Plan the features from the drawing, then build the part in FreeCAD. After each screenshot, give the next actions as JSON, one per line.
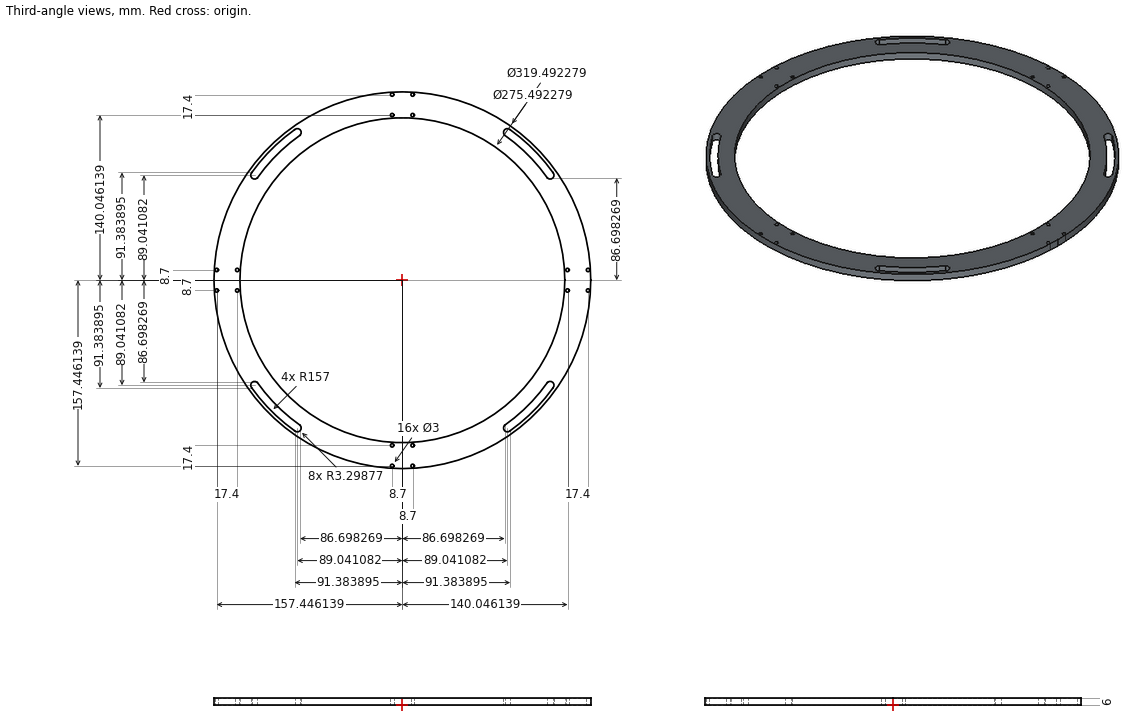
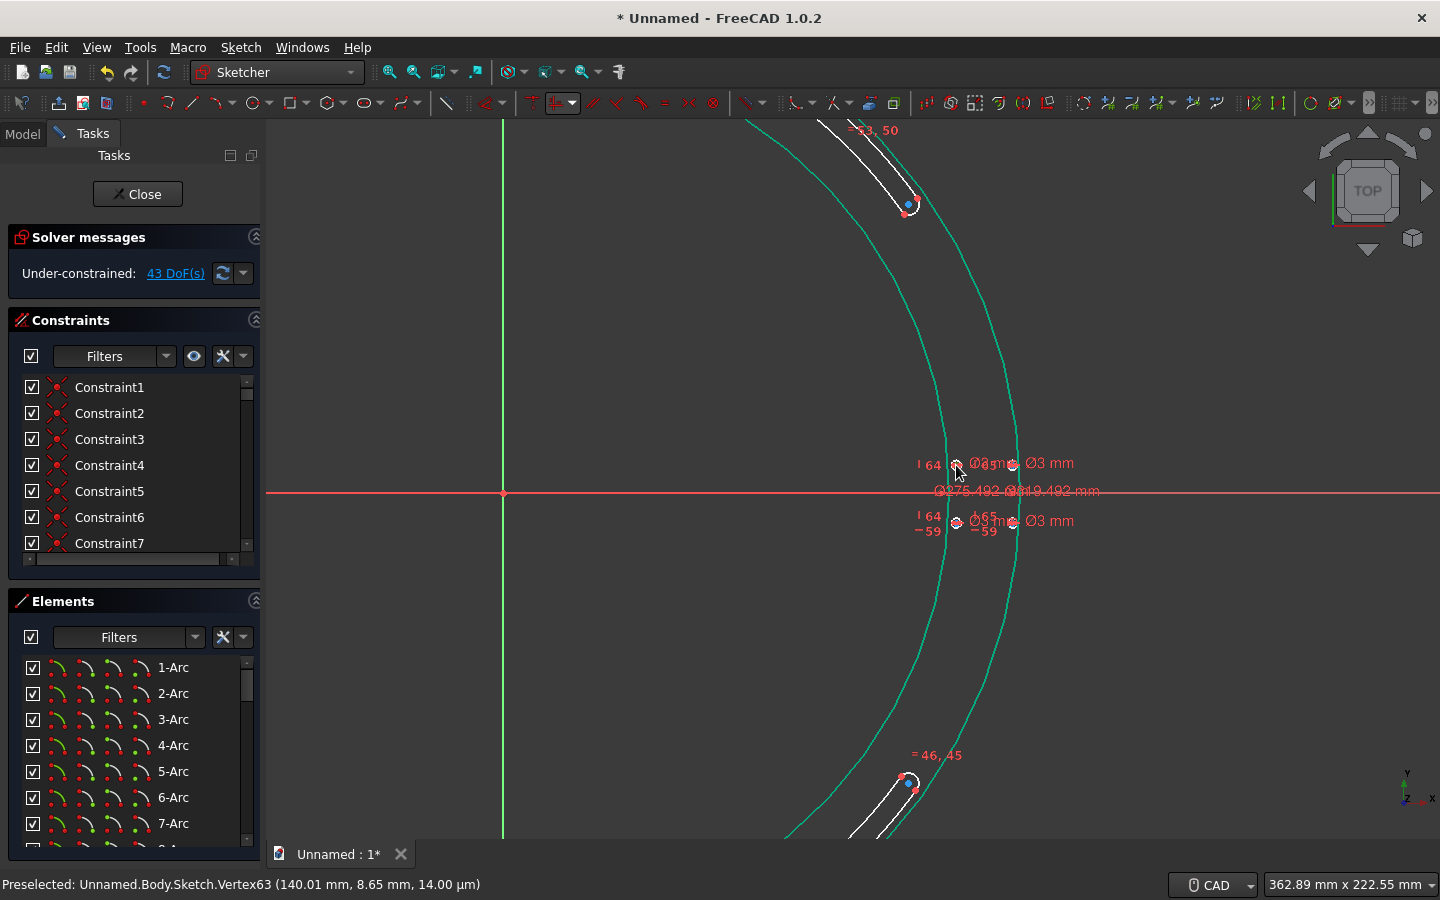
{"action": "left_click", "coordinate": [1013, 465]}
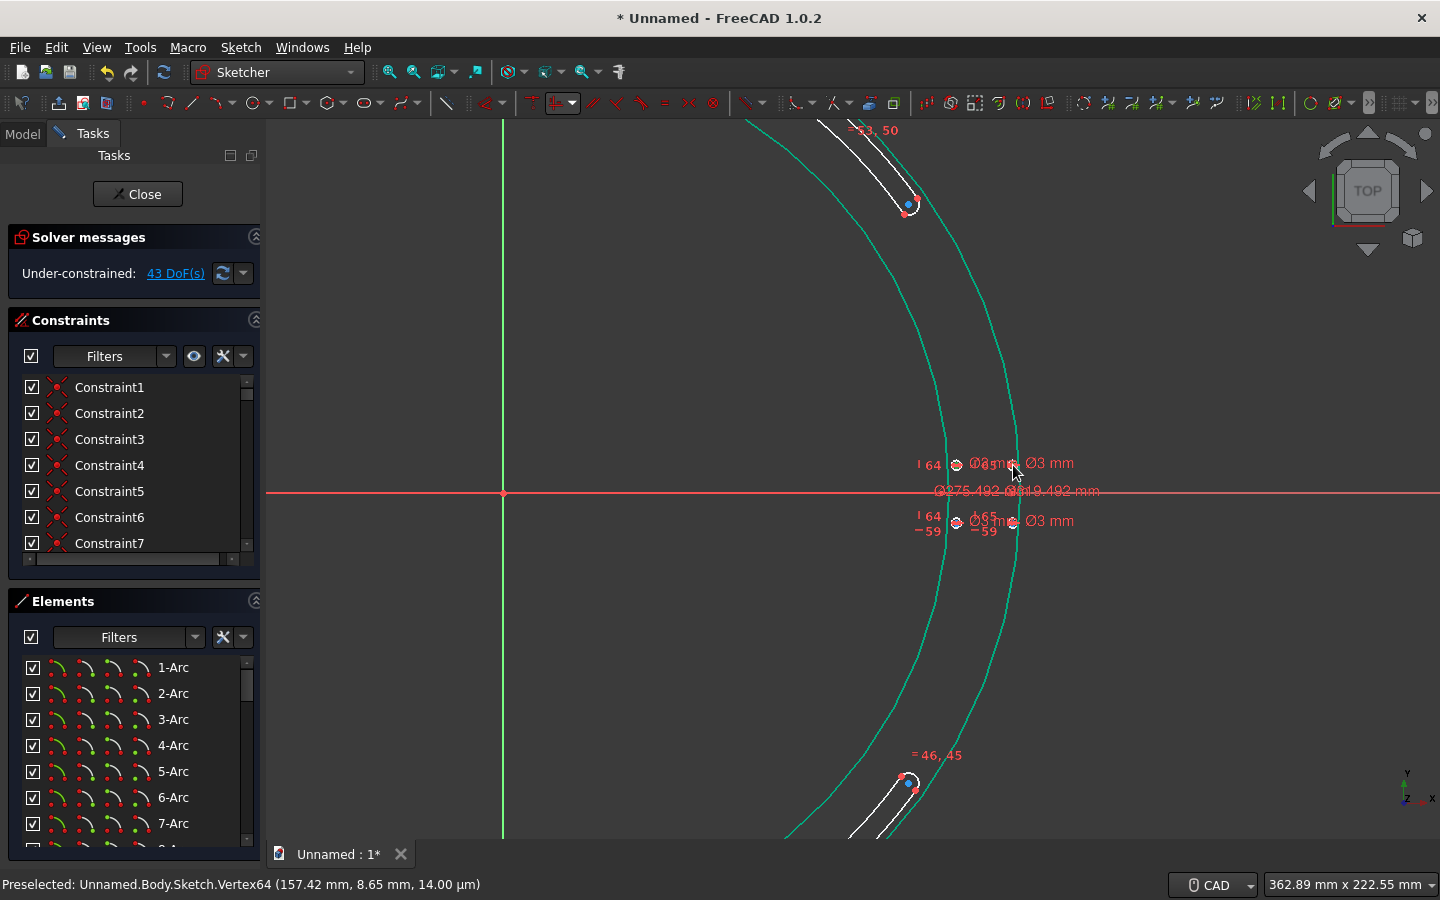
{"action": "key", "text": "h"}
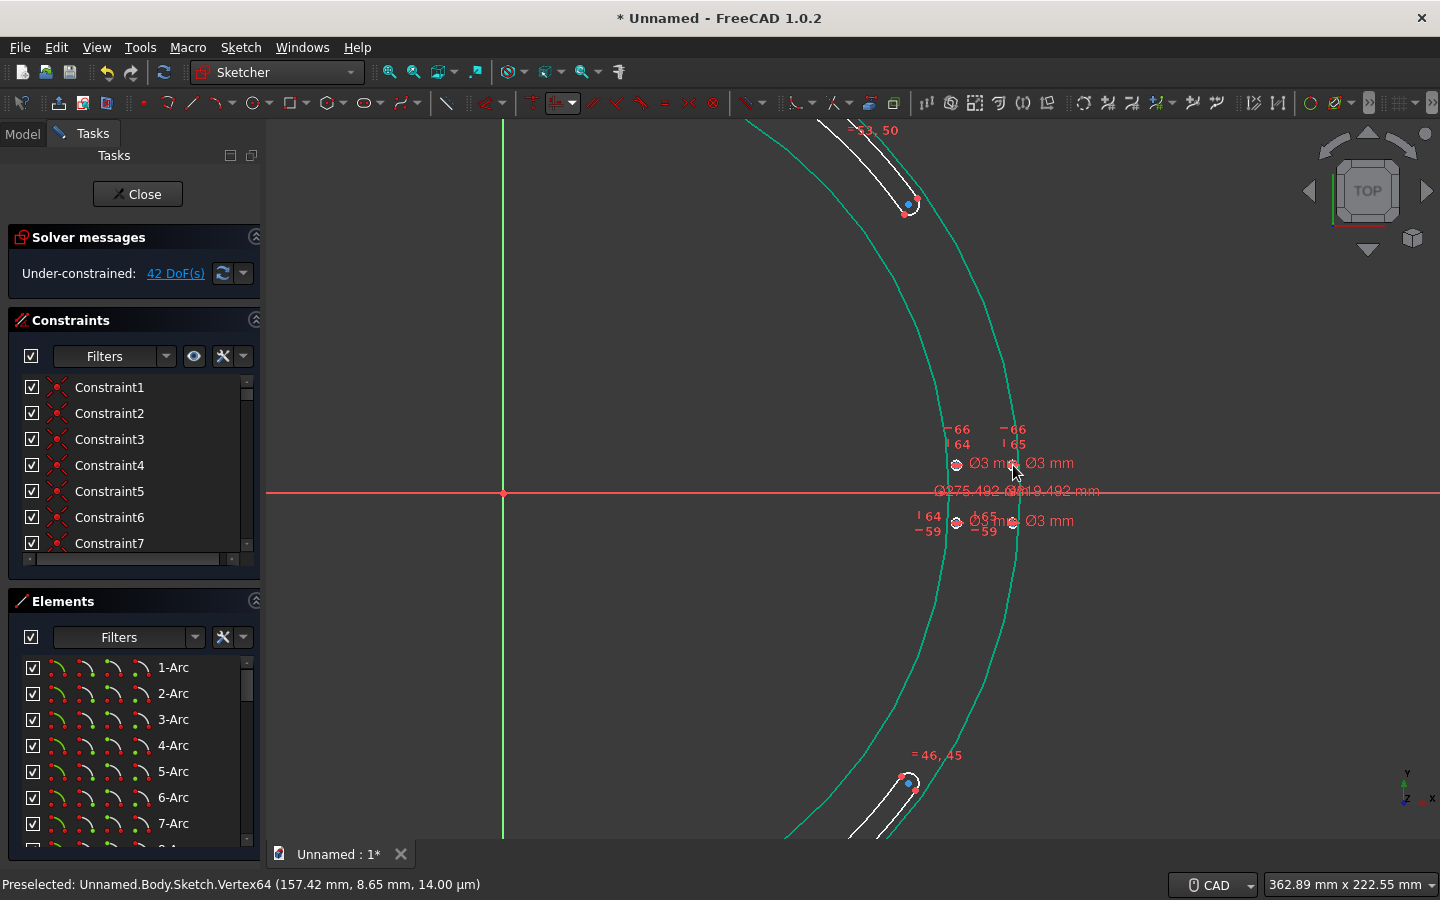
{"action": "scroll", "coordinate": [1014, 467], "scroll_direction": "down", "scroll_amount": 4}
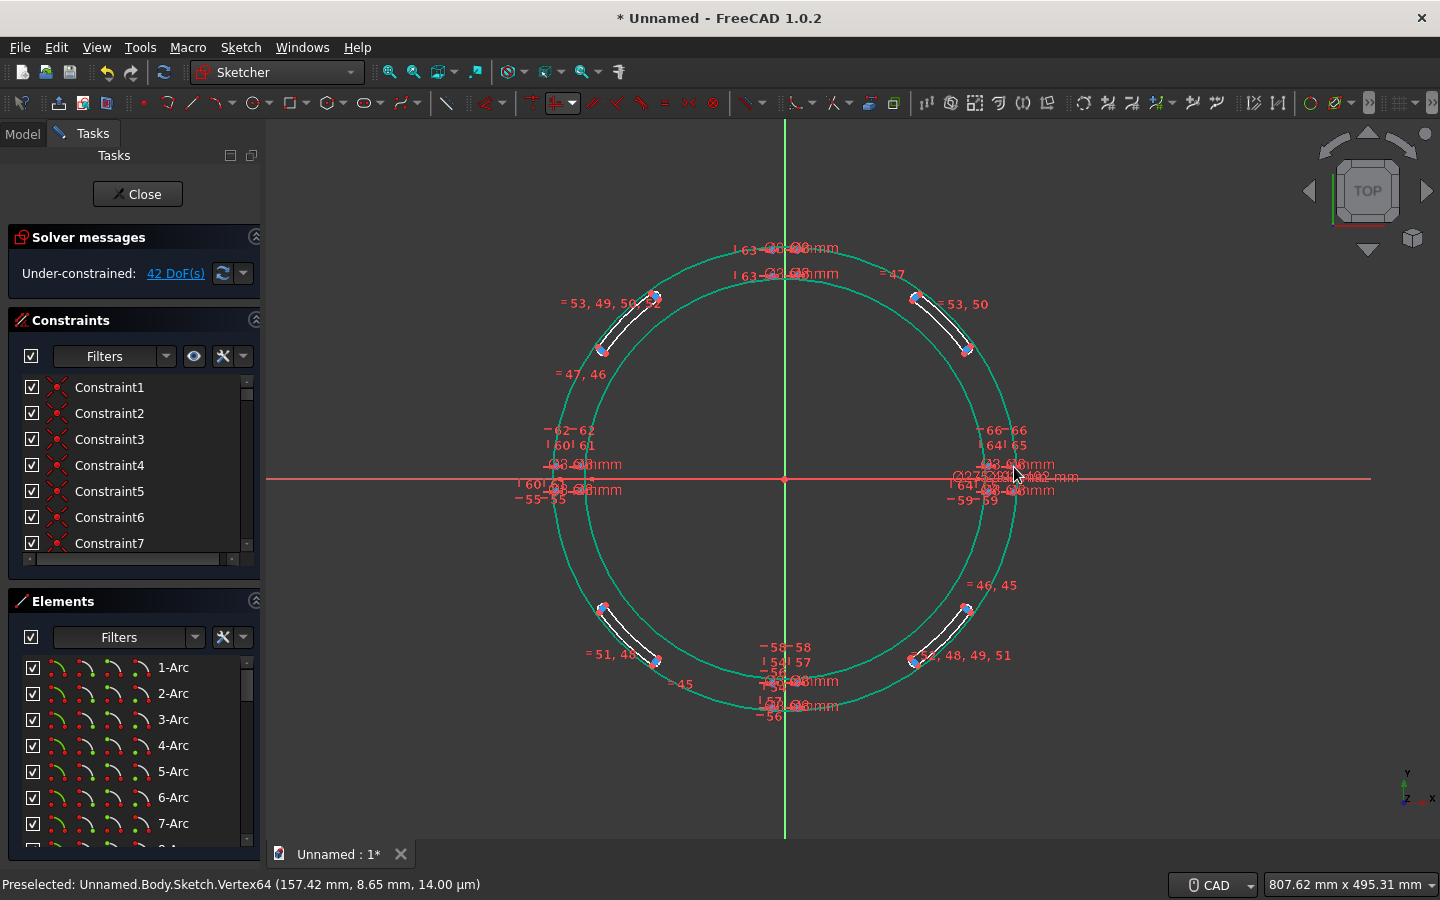
{"action": "left_click", "coordinate": [772, 276]}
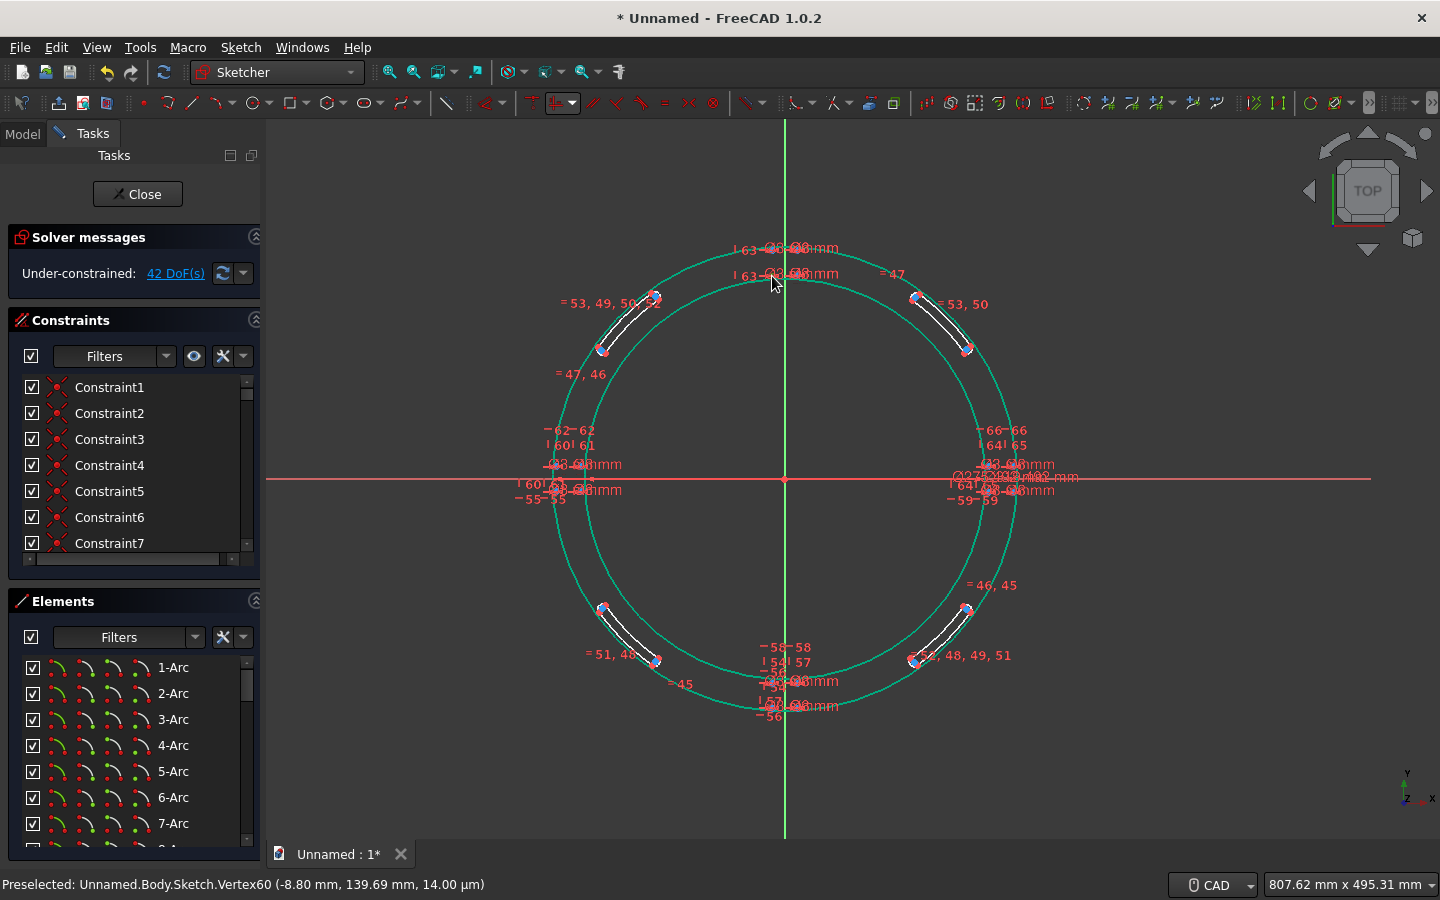
{"action": "left_click", "coordinate": [798, 276]}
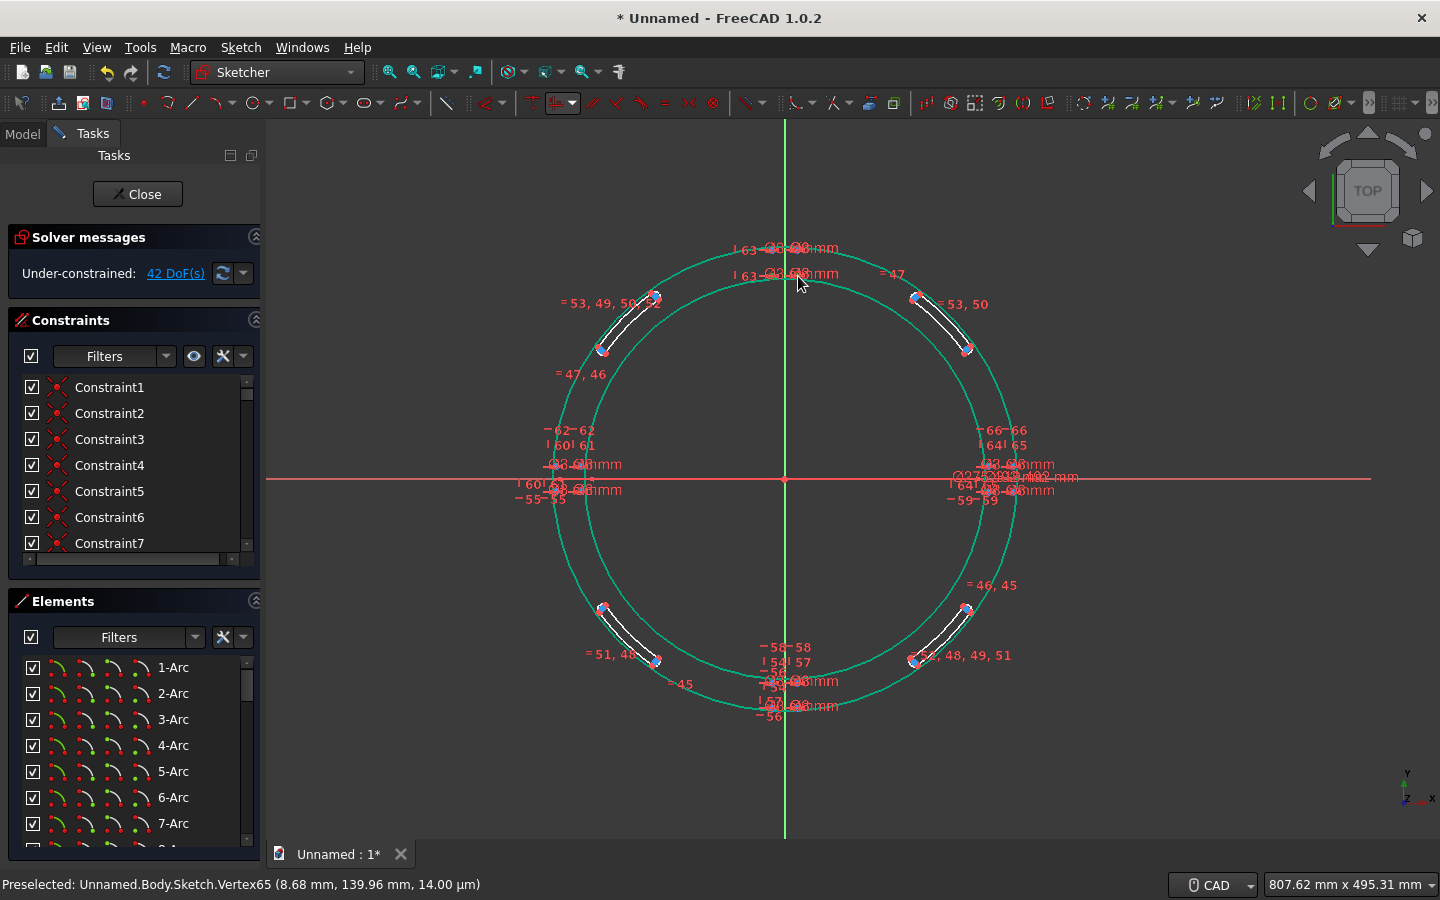
{"action": "left_click", "coordinate": [574, 104]}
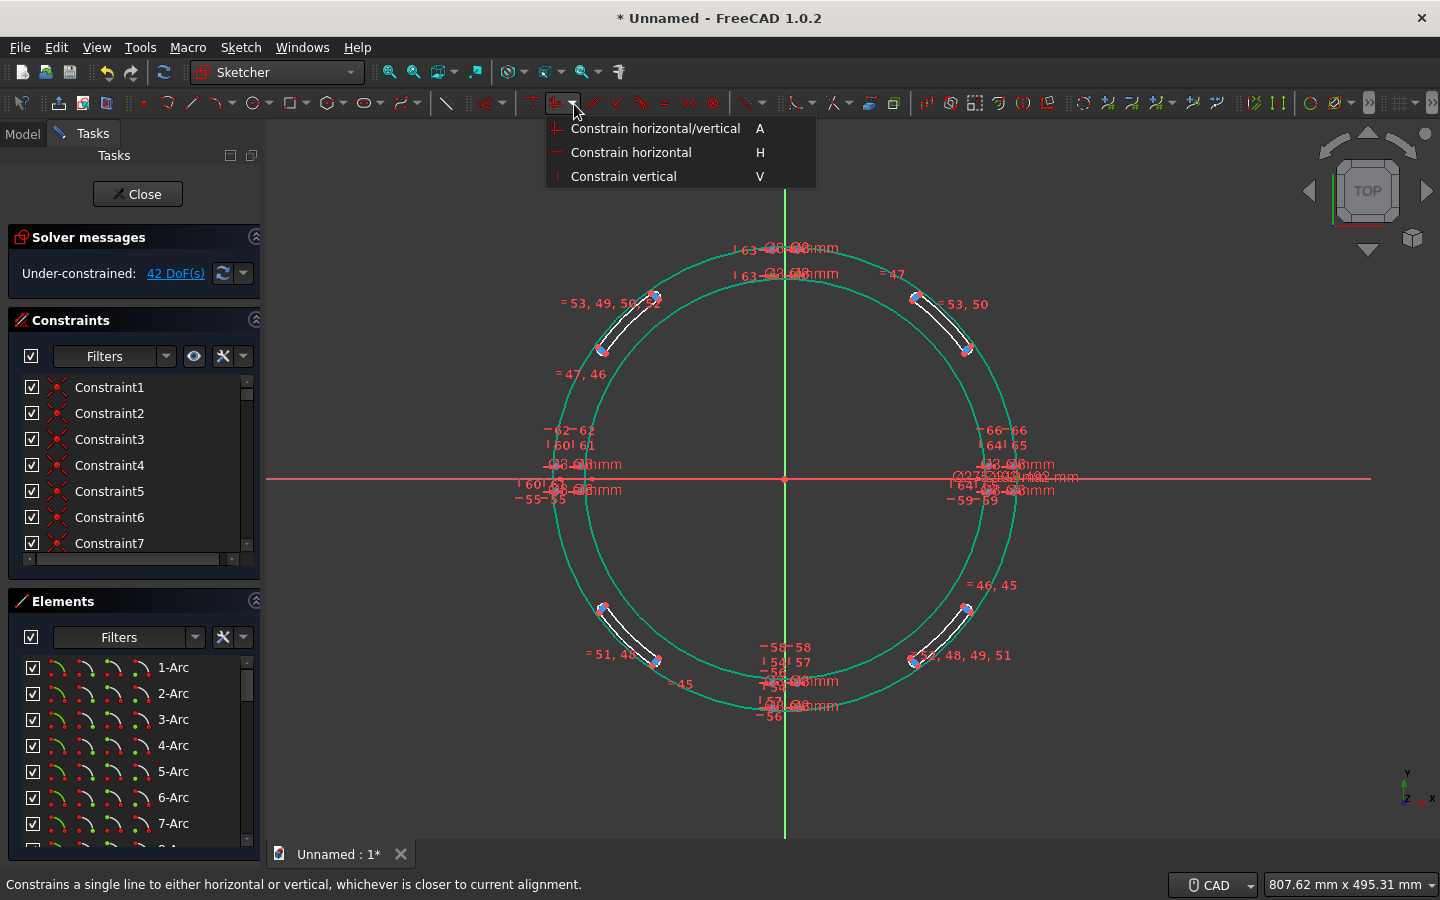
{"action": "left_click", "coordinate": [681, 152]}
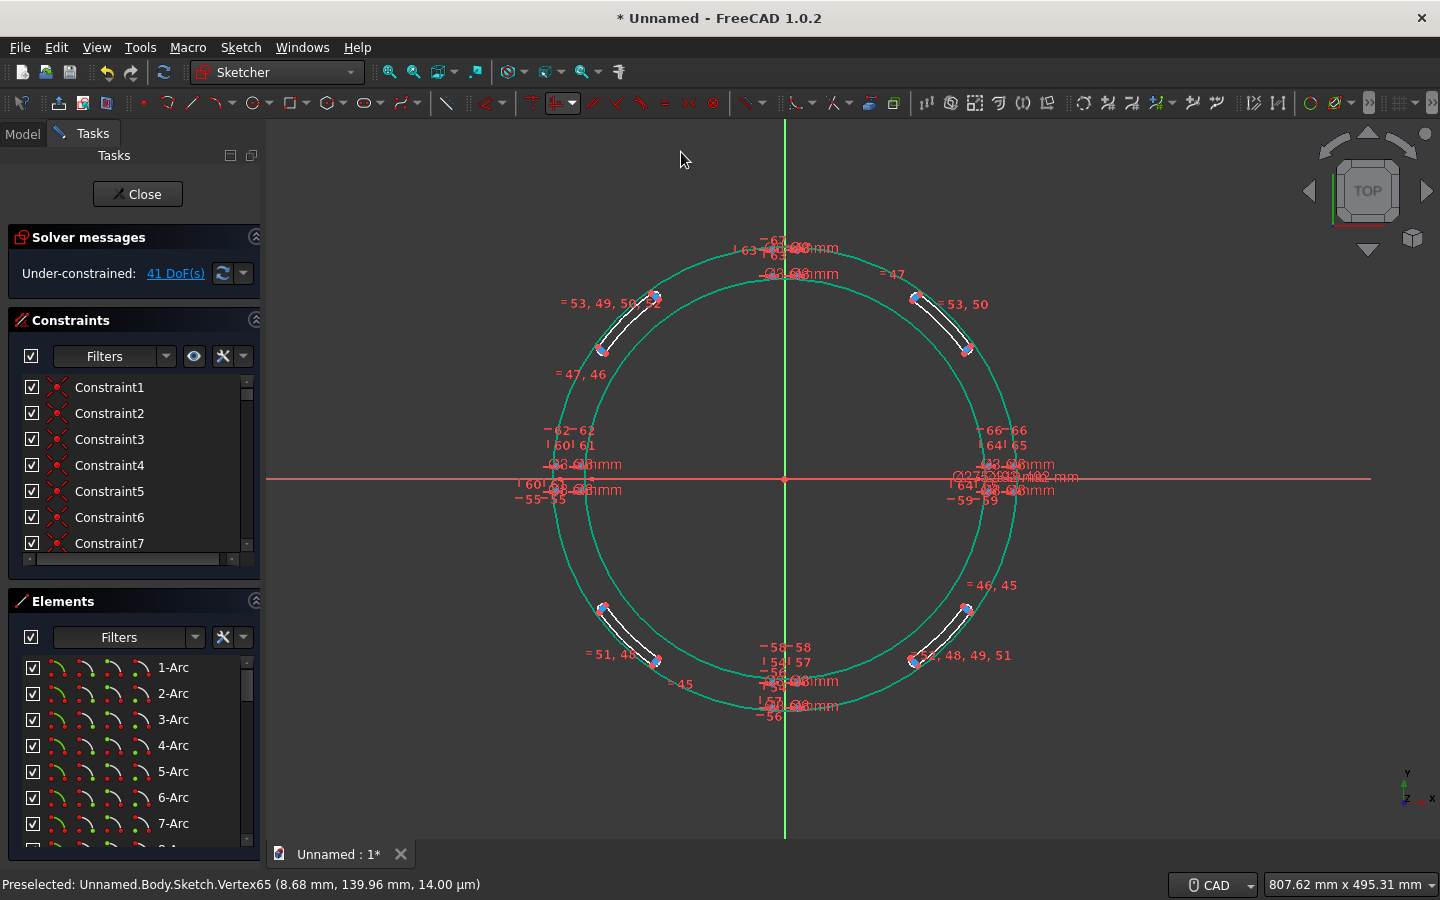
{"action": "left_click", "coordinate": [798, 276]}